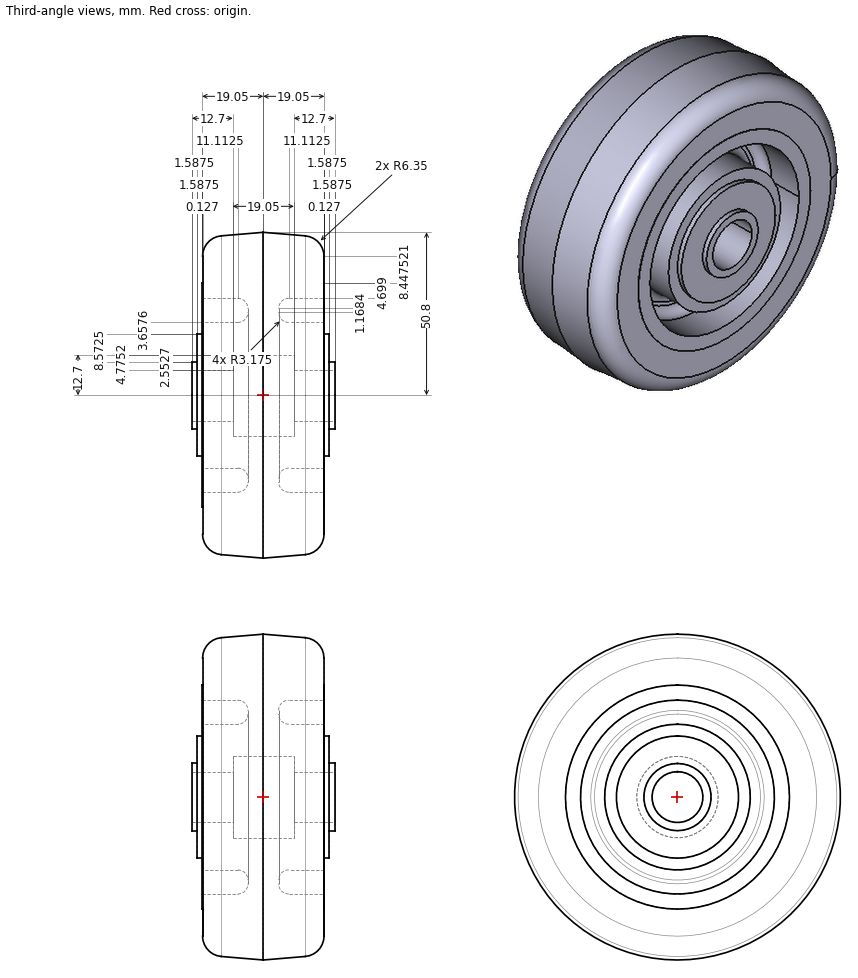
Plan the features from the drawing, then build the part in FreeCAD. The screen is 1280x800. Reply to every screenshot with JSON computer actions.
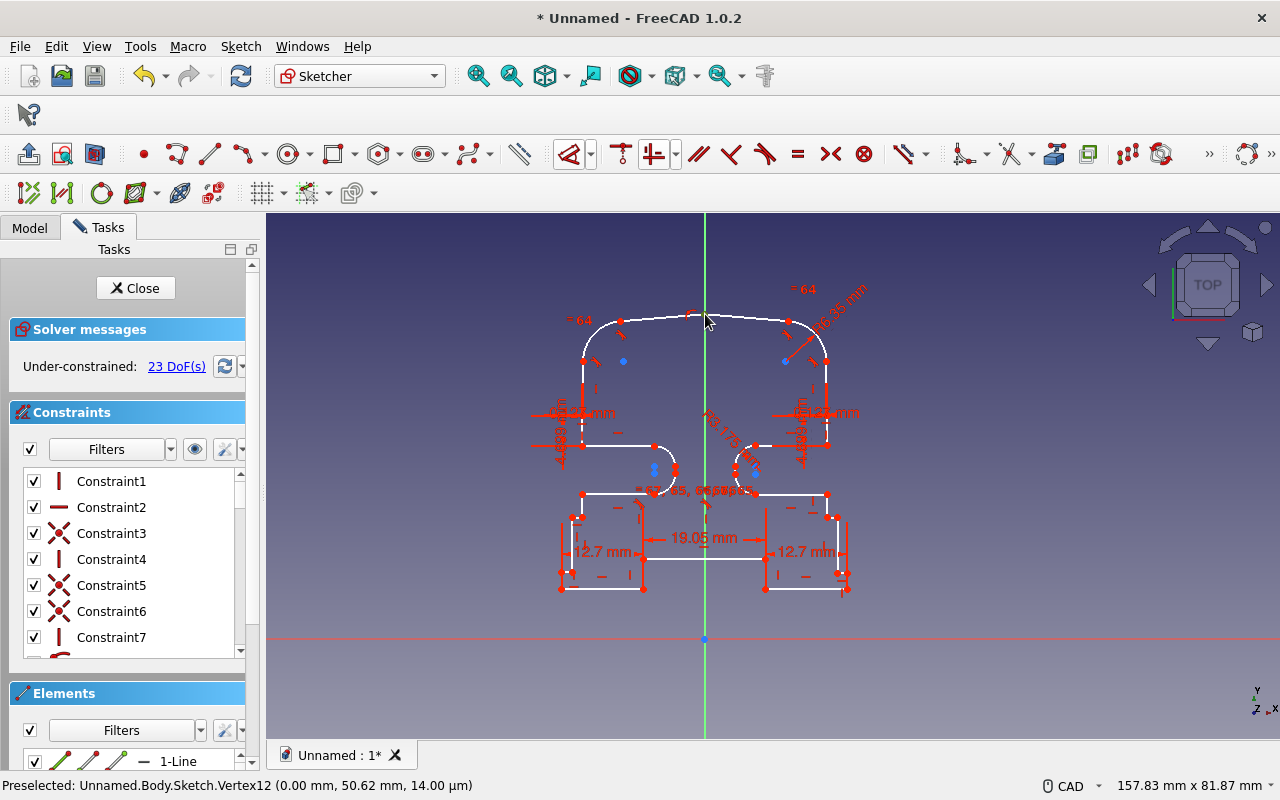
{"action": "key", "text": "i"}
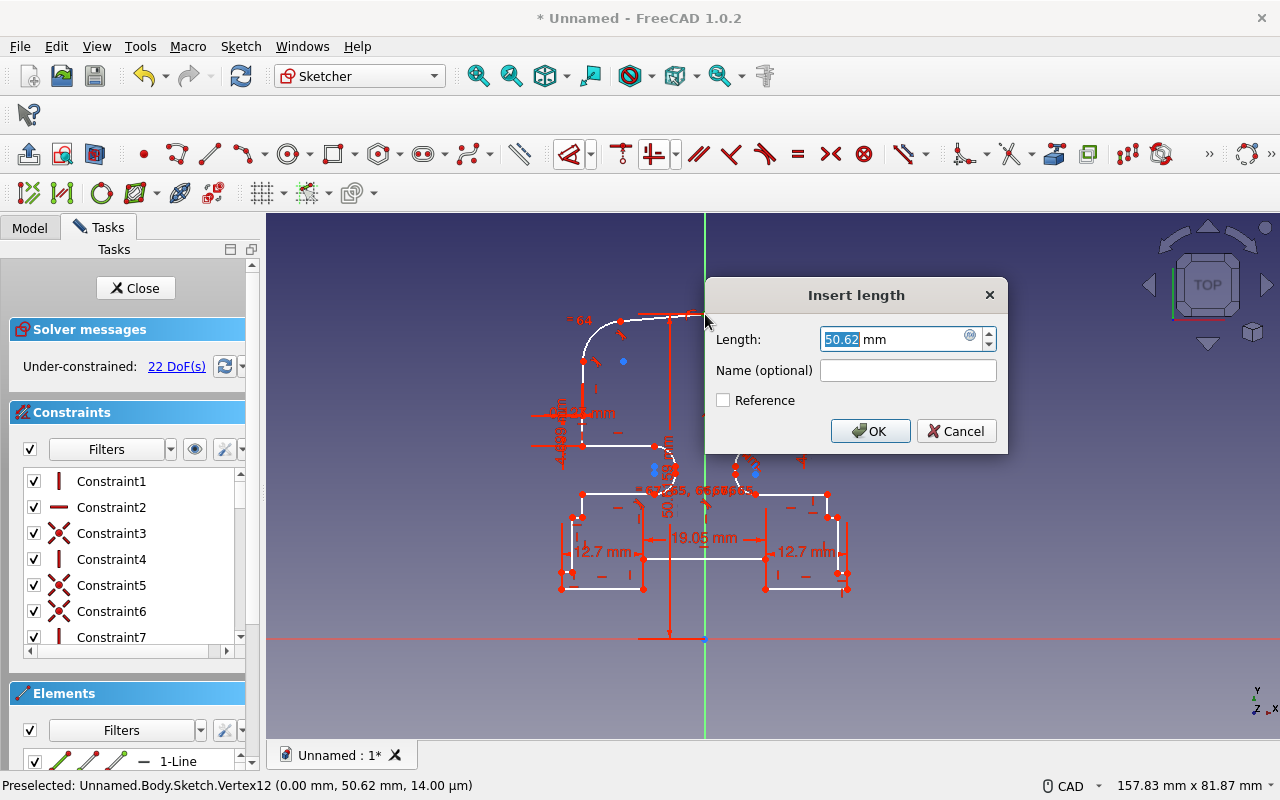
{"action": "type", "text": "50.8"}
{"action": "key", "text": "Return"}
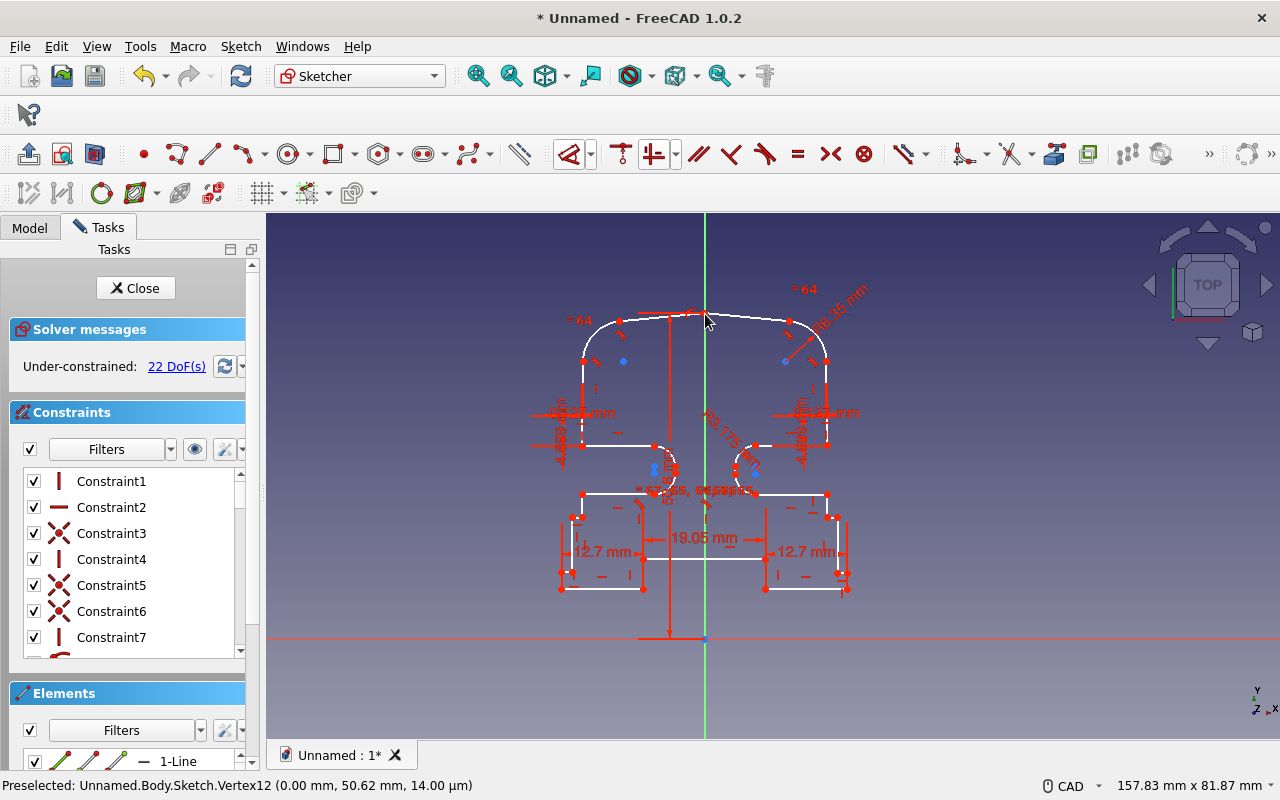
{"action": "left_click", "coordinate": [643, 559]}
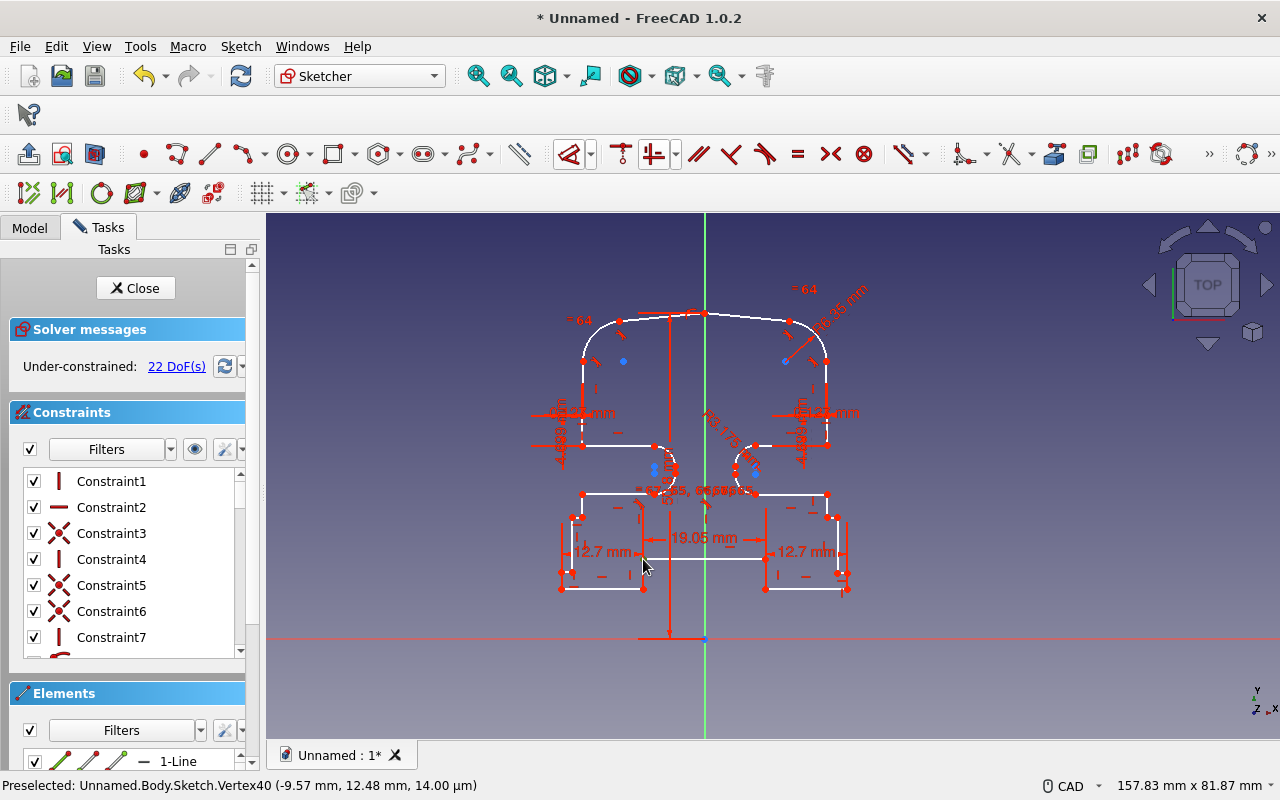
{"action": "left_click", "coordinate": [590, 154]}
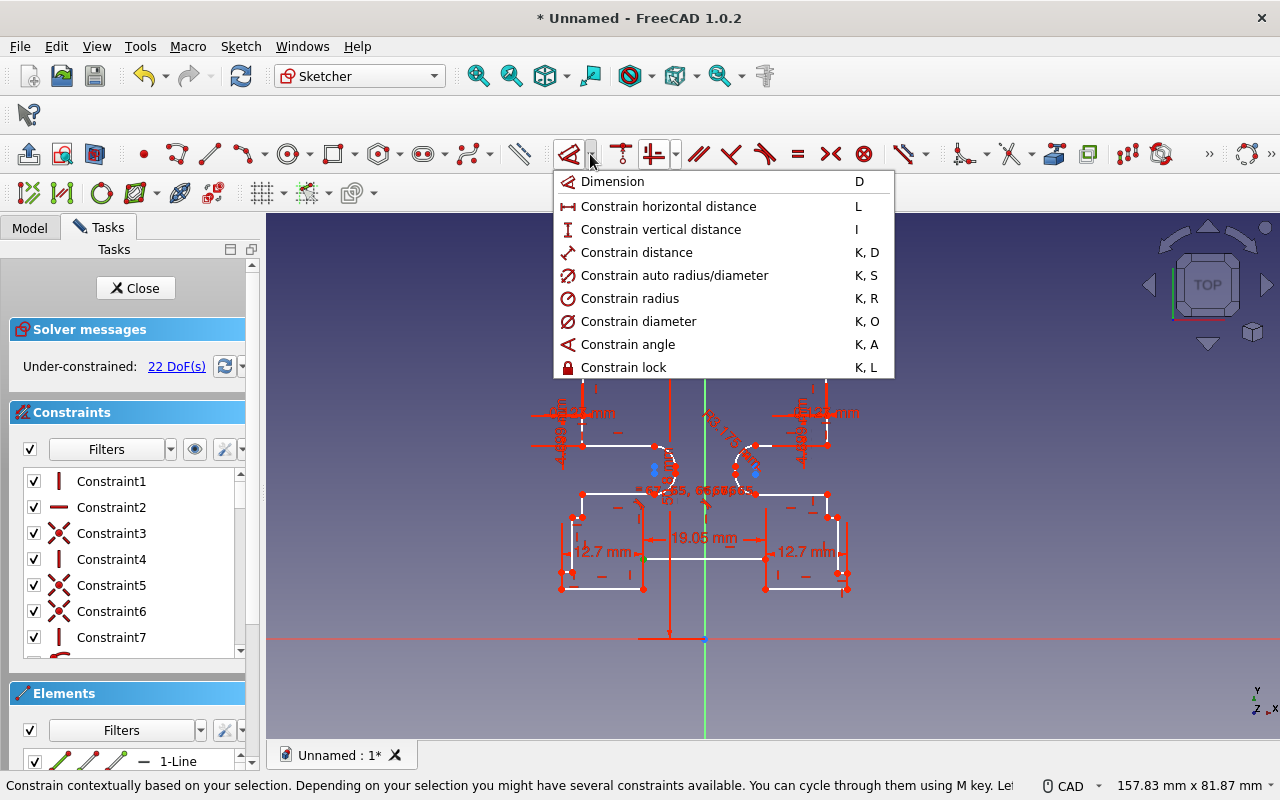
{"action": "left_click", "coordinate": [724, 230]}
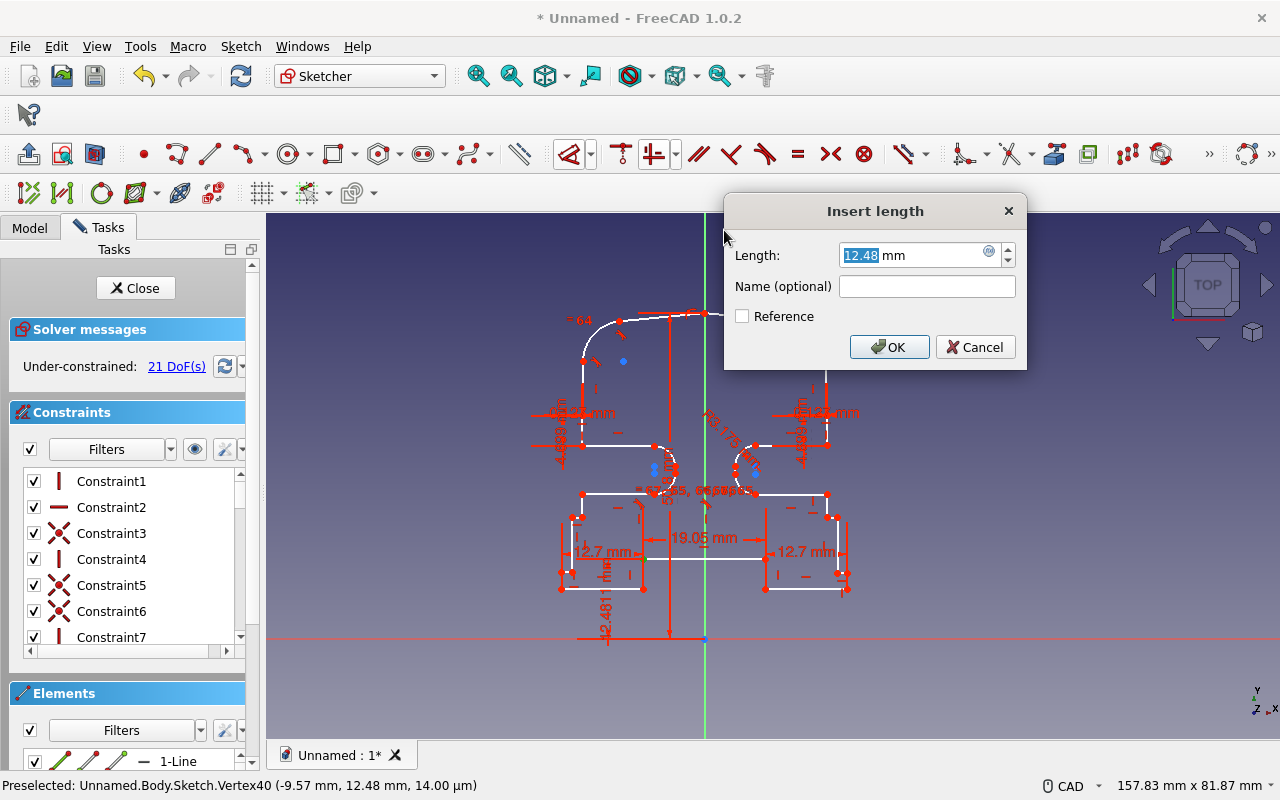
{"action": "type", "text": "12.7"}
{"action": "key", "text": "Return"}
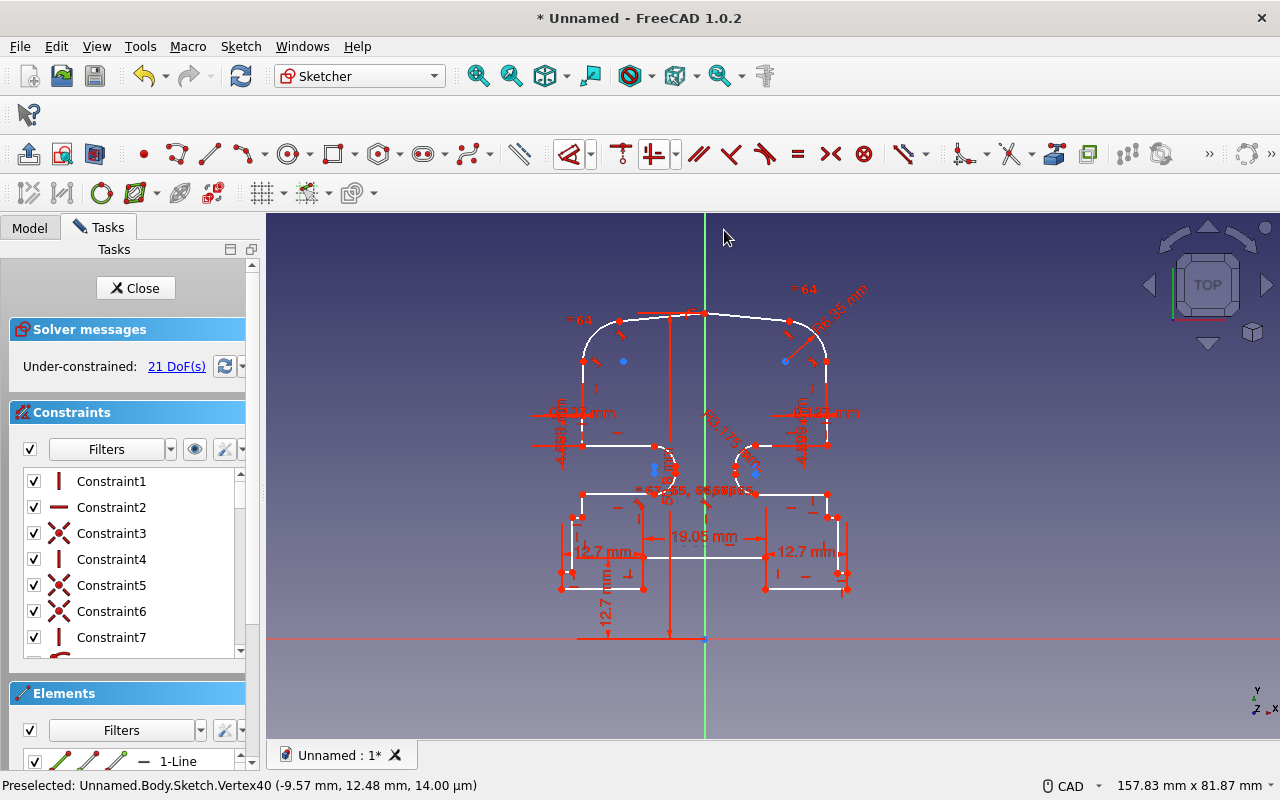
{"action": "scroll", "coordinate": [735, 470], "scroll_direction": "up", "scroll_amount": 9}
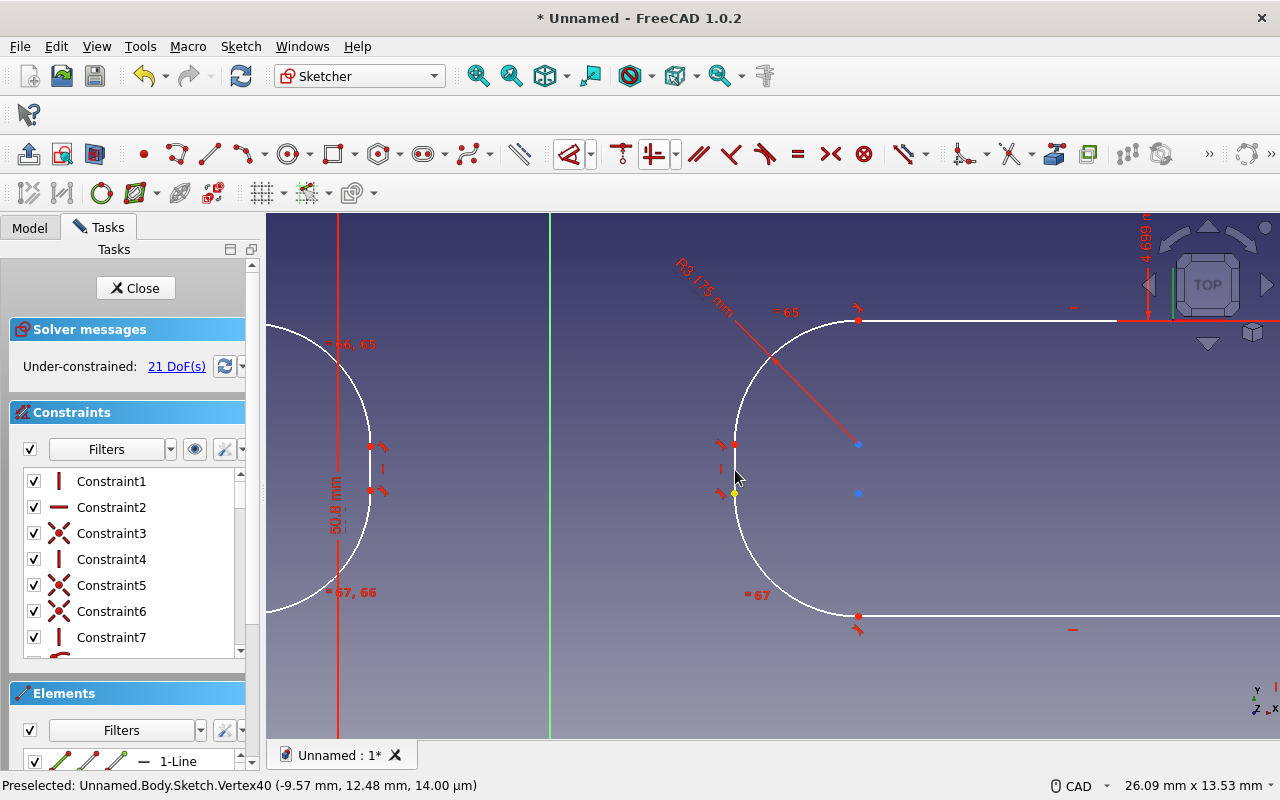
{"action": "left_click", "coordinate": [735, 469]}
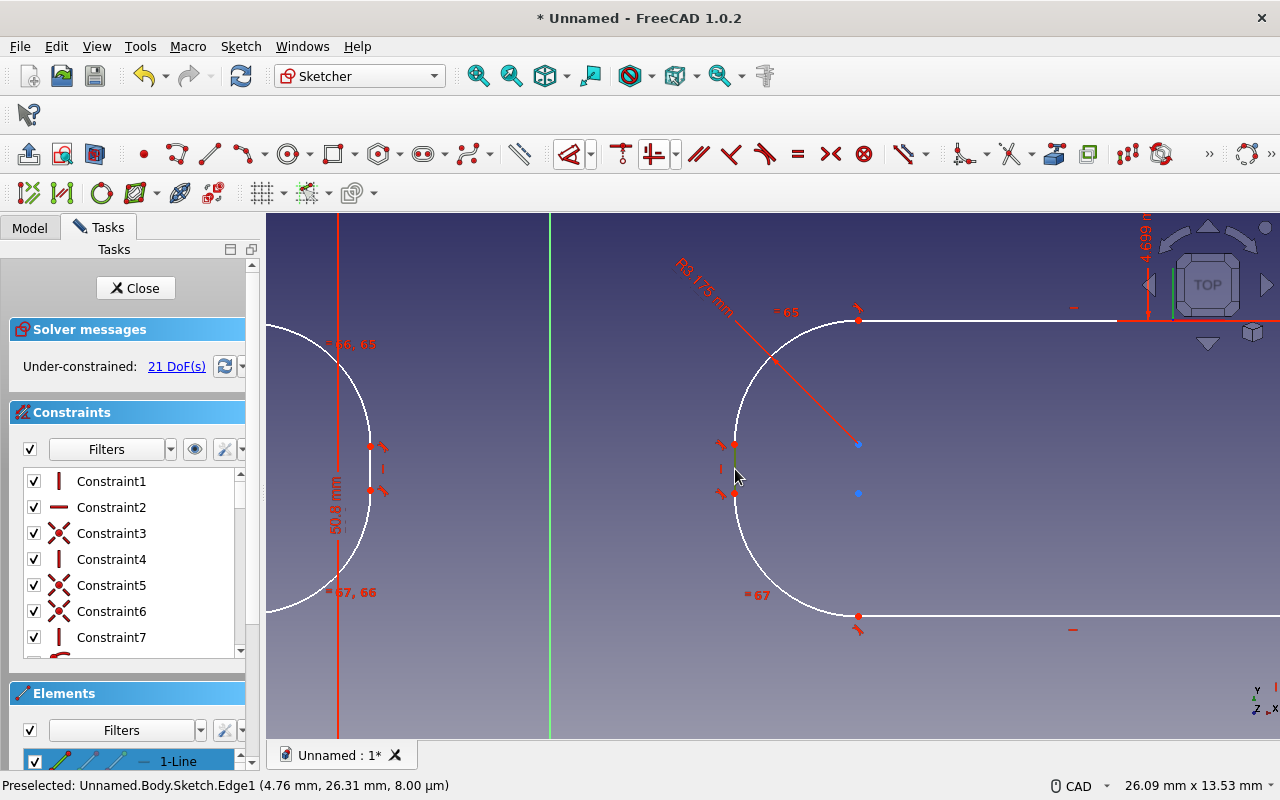
{"action": "left_click", "coordinate": [590, 154]}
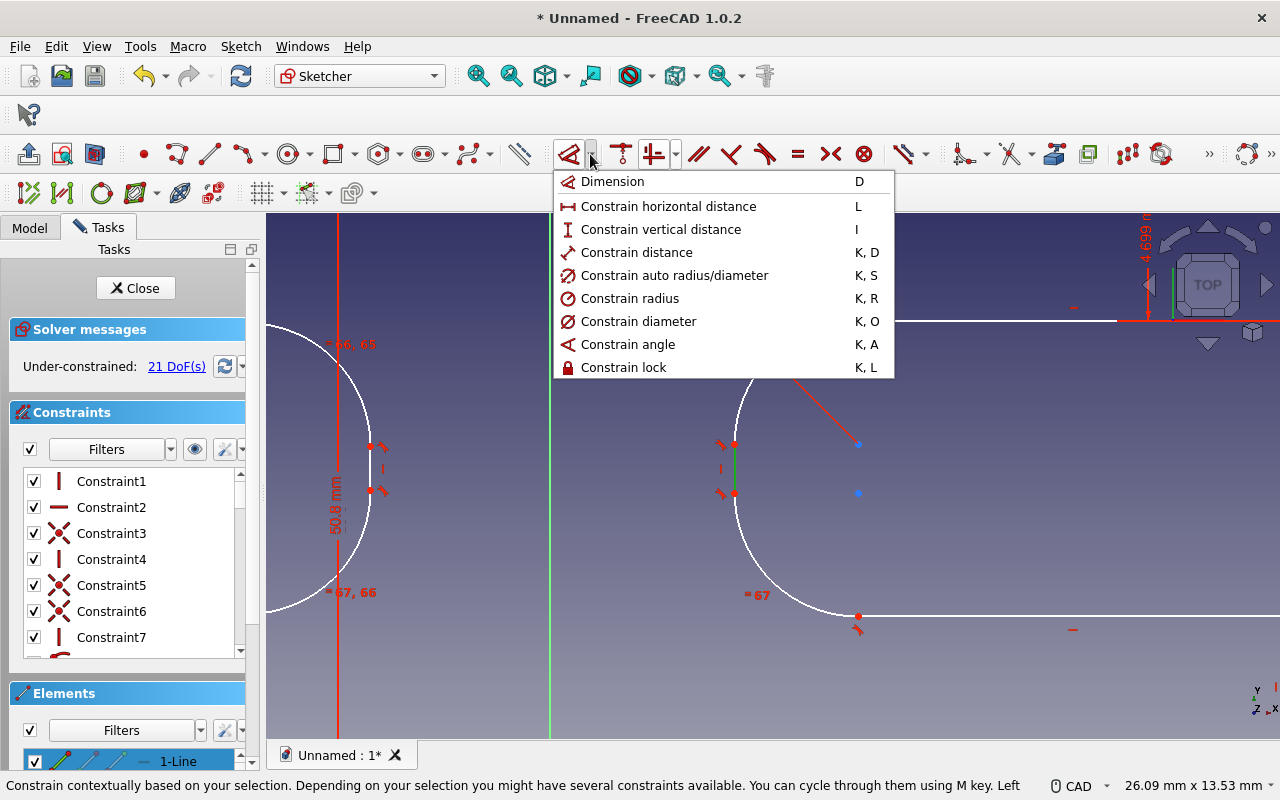
{"action": "left_click", "coordinate": [724, 230]}